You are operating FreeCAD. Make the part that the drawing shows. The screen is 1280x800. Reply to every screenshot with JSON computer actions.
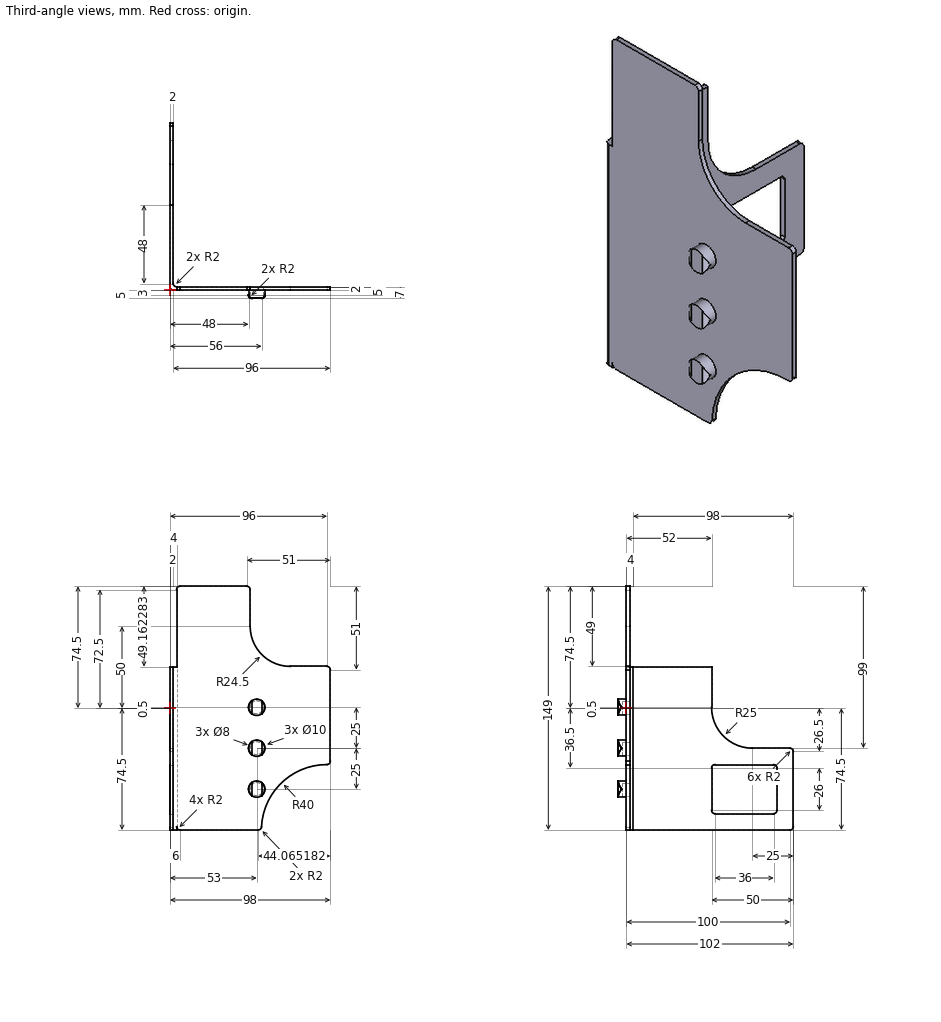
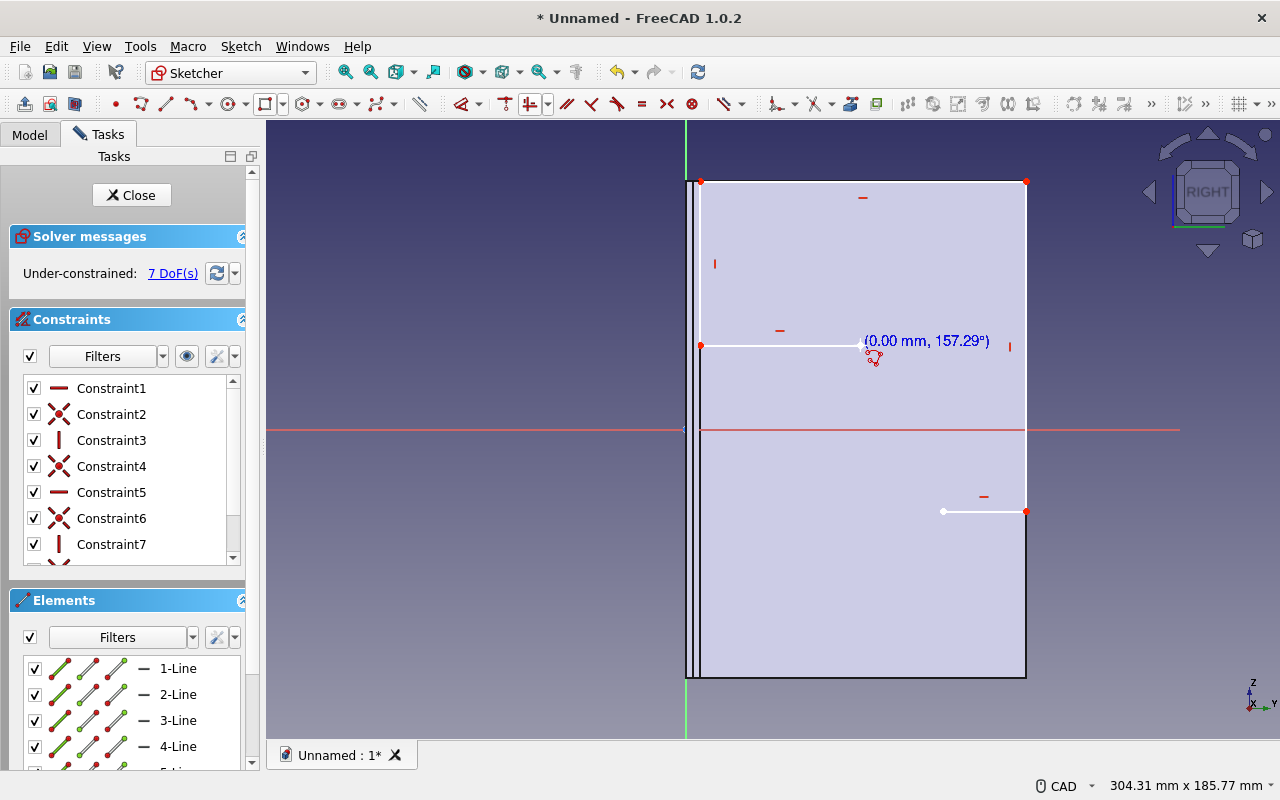
{"action": "scroll", "coordinate": [860, 428], "scroll_direction": "up", "scroll_amount": 12}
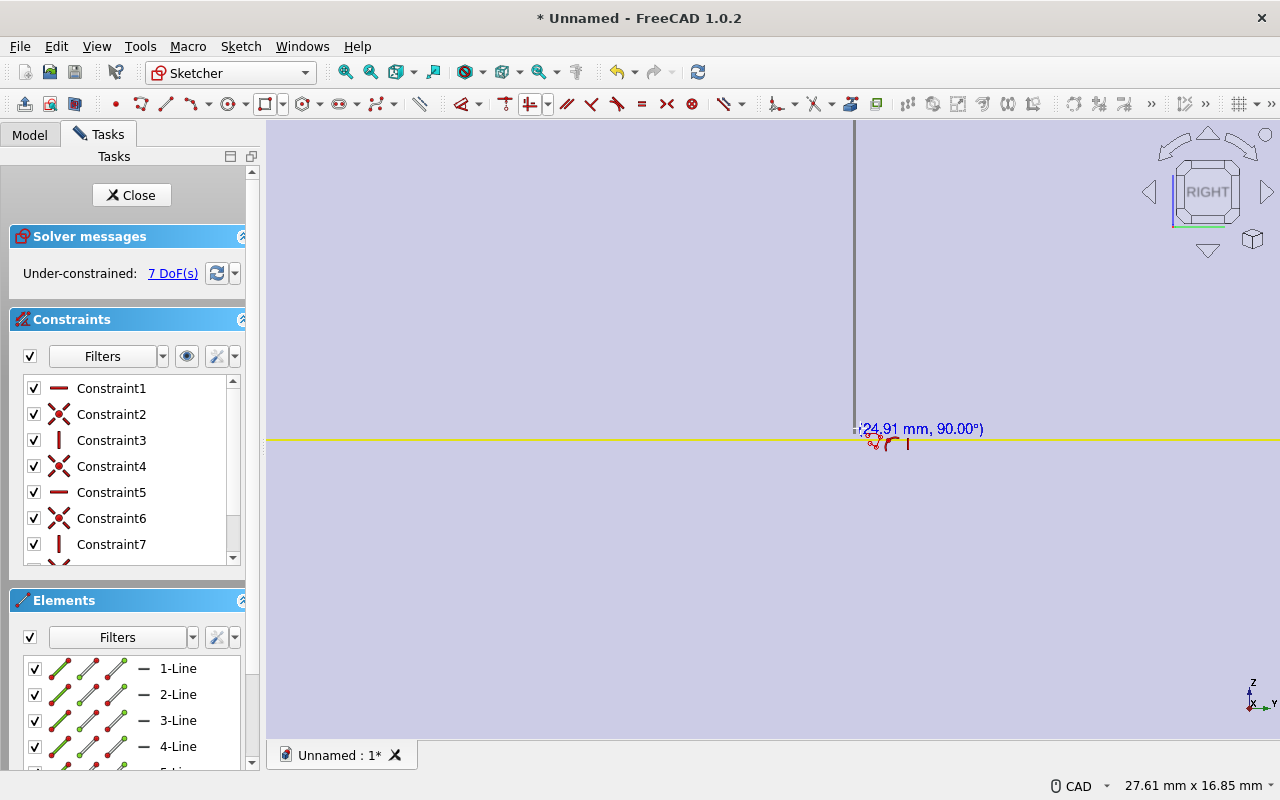
{"action": "left_click", "coordinate": [854, 421]}
{"action": "right_click", "coordinate": [854, 421]}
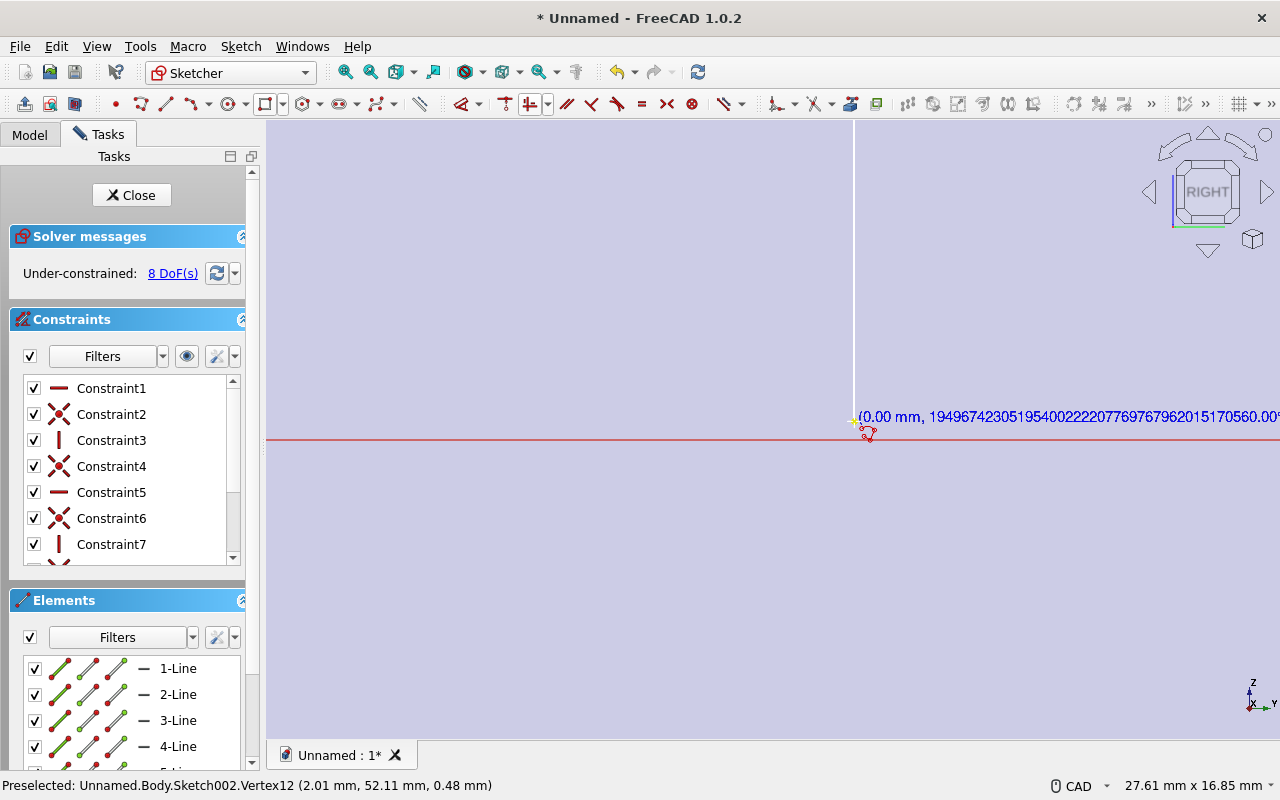
{"action": "key", "text": "g 3 a"}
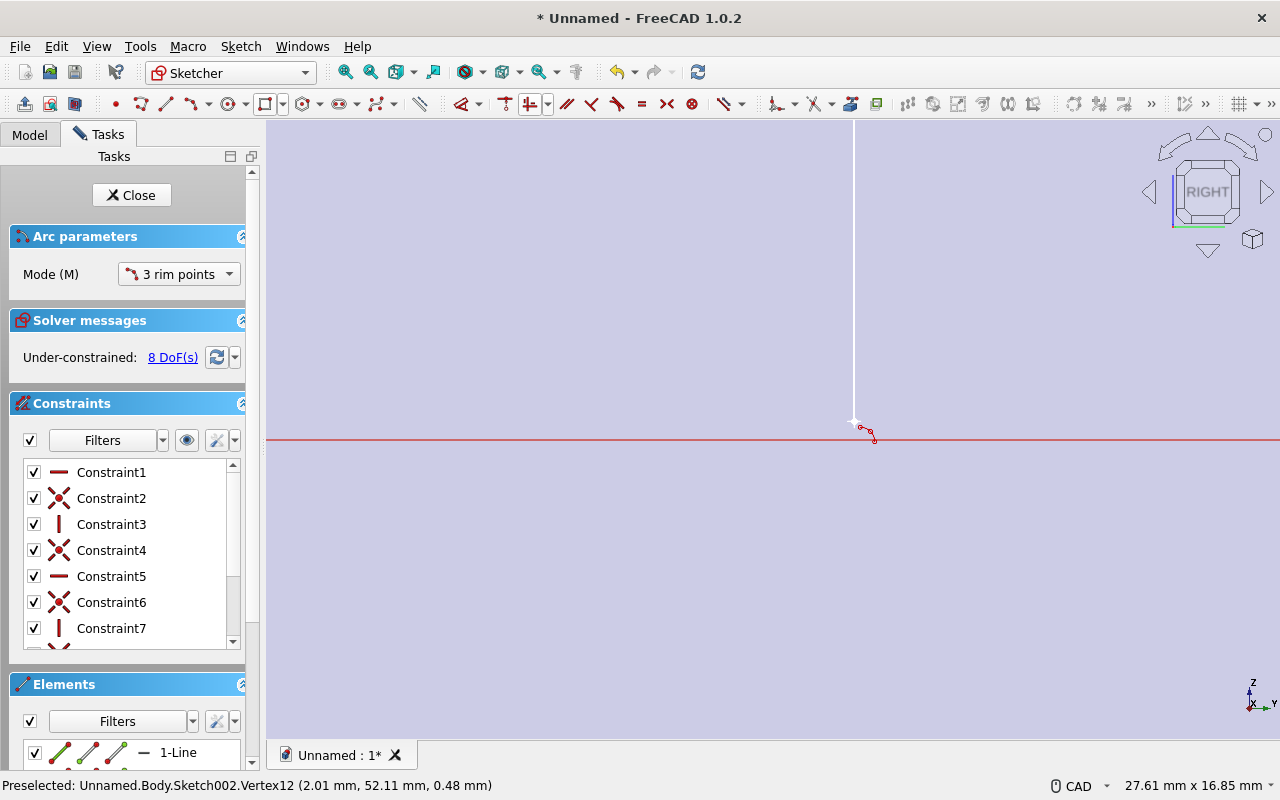
{"action": "left_click", "coordinate": [854, 422]}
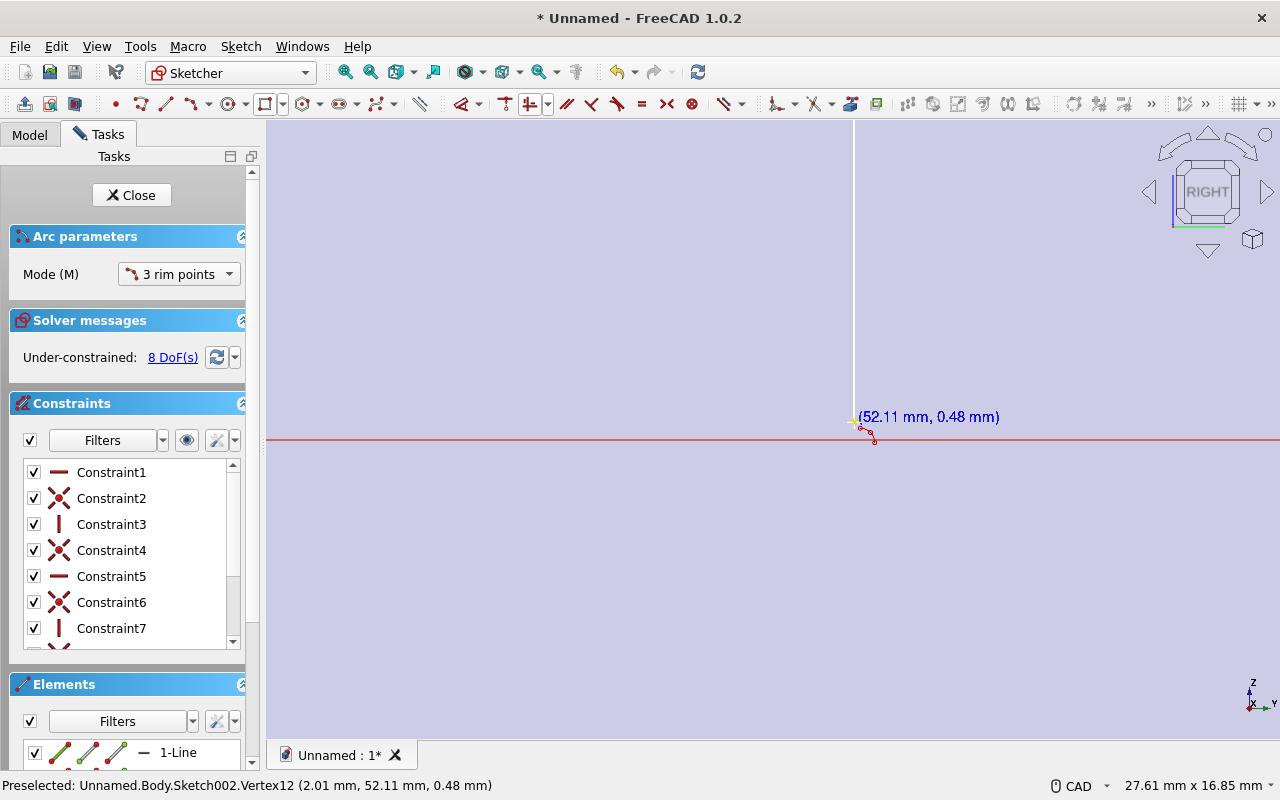
{"action": "scroll", "coordinate": [691, 543], "scroll_direction": "down", "scroll_amount": 11}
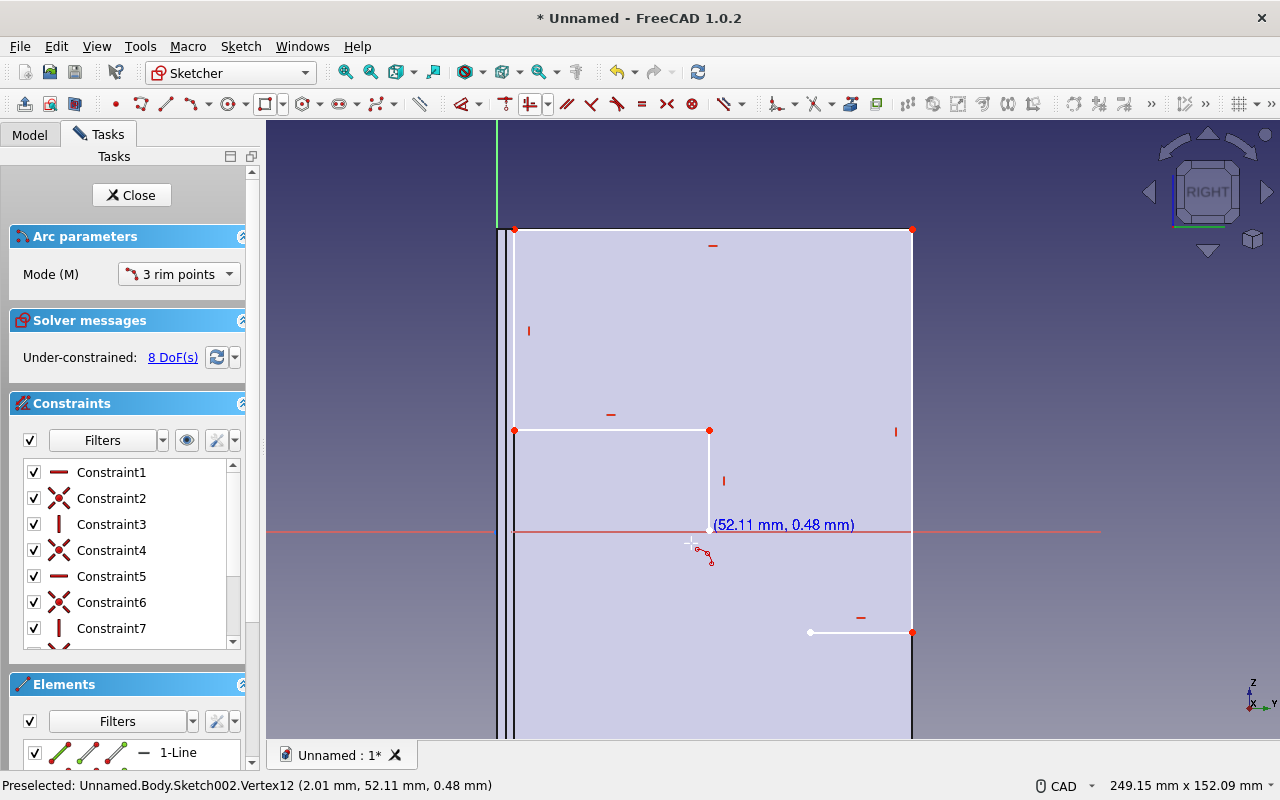
{"action": "left_click", "coordinate": [811, 633]}
{"action": "left_click", "coordinate": [739, 602]}
{"action": "key", "text": "Escape"}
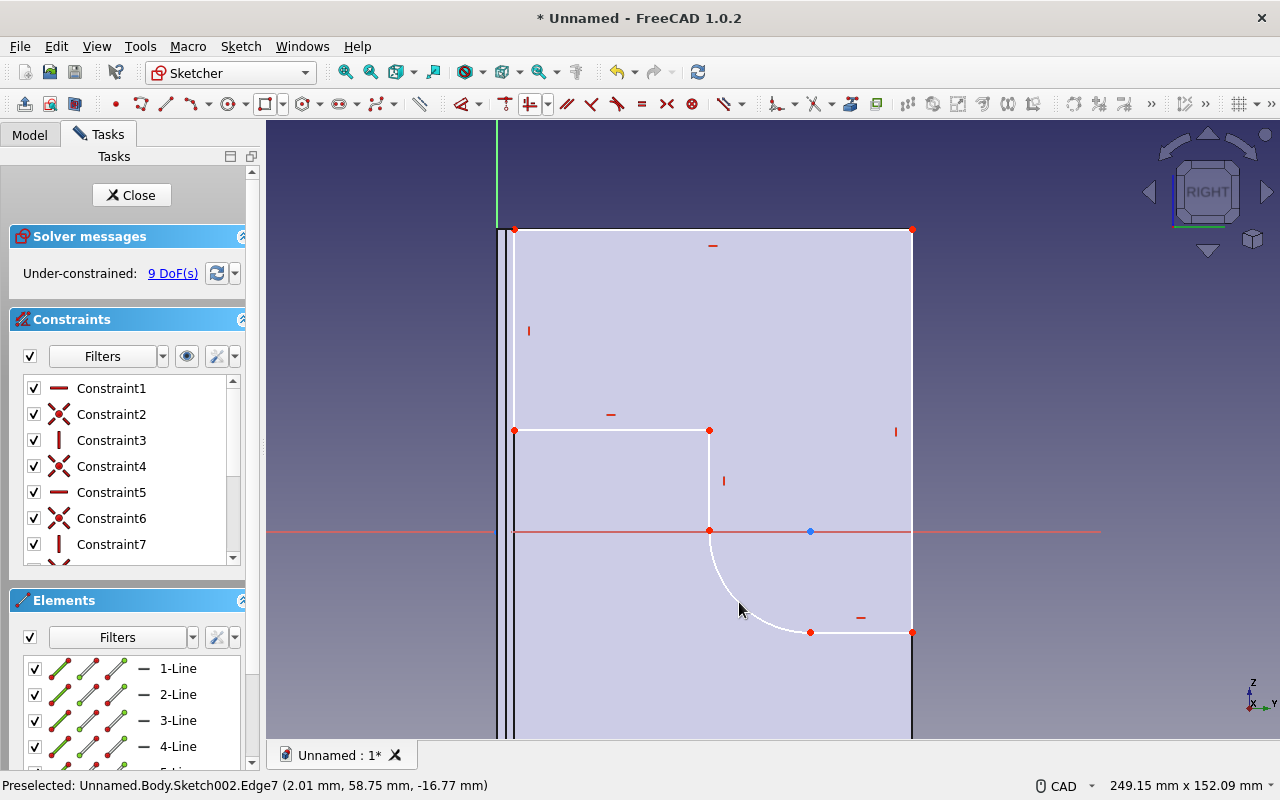
{"action": "left_click", "coordinate": [841, 633]}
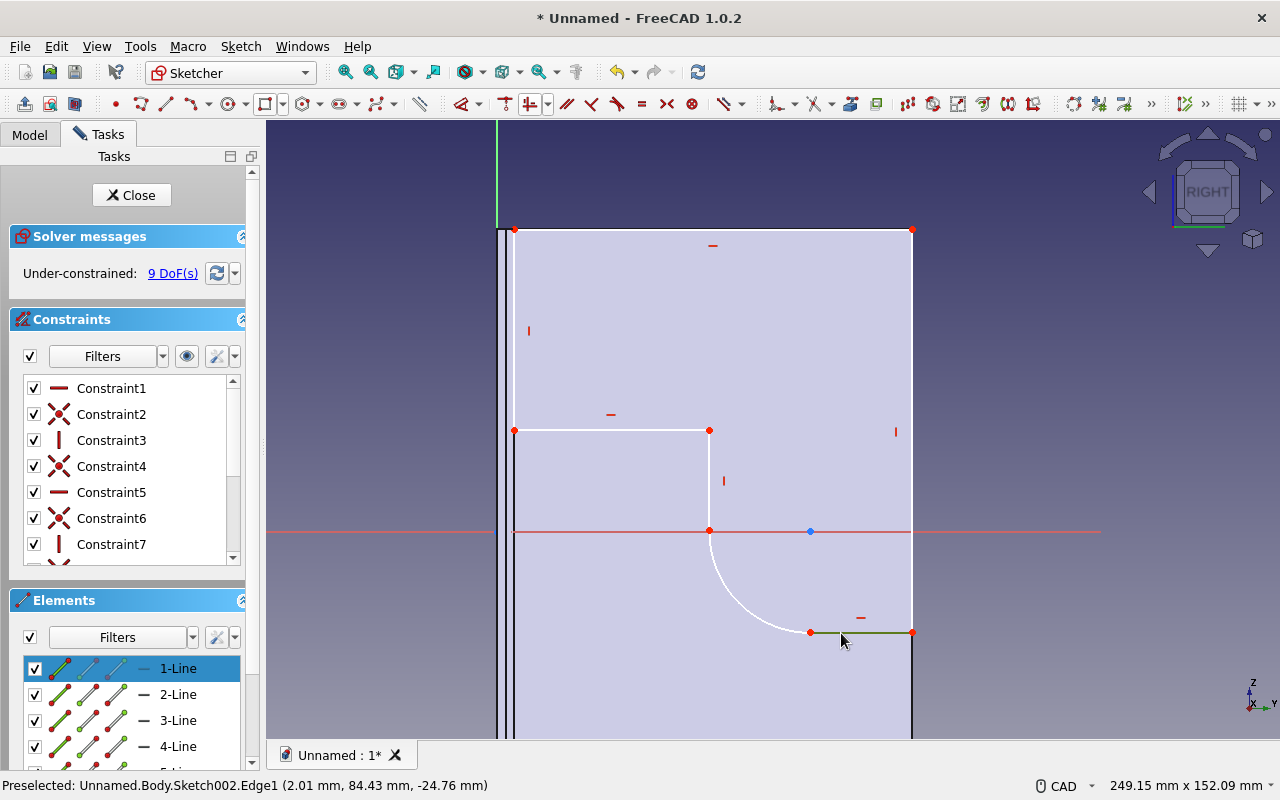
{"action": "left_click", "coordinate": [720, 577]}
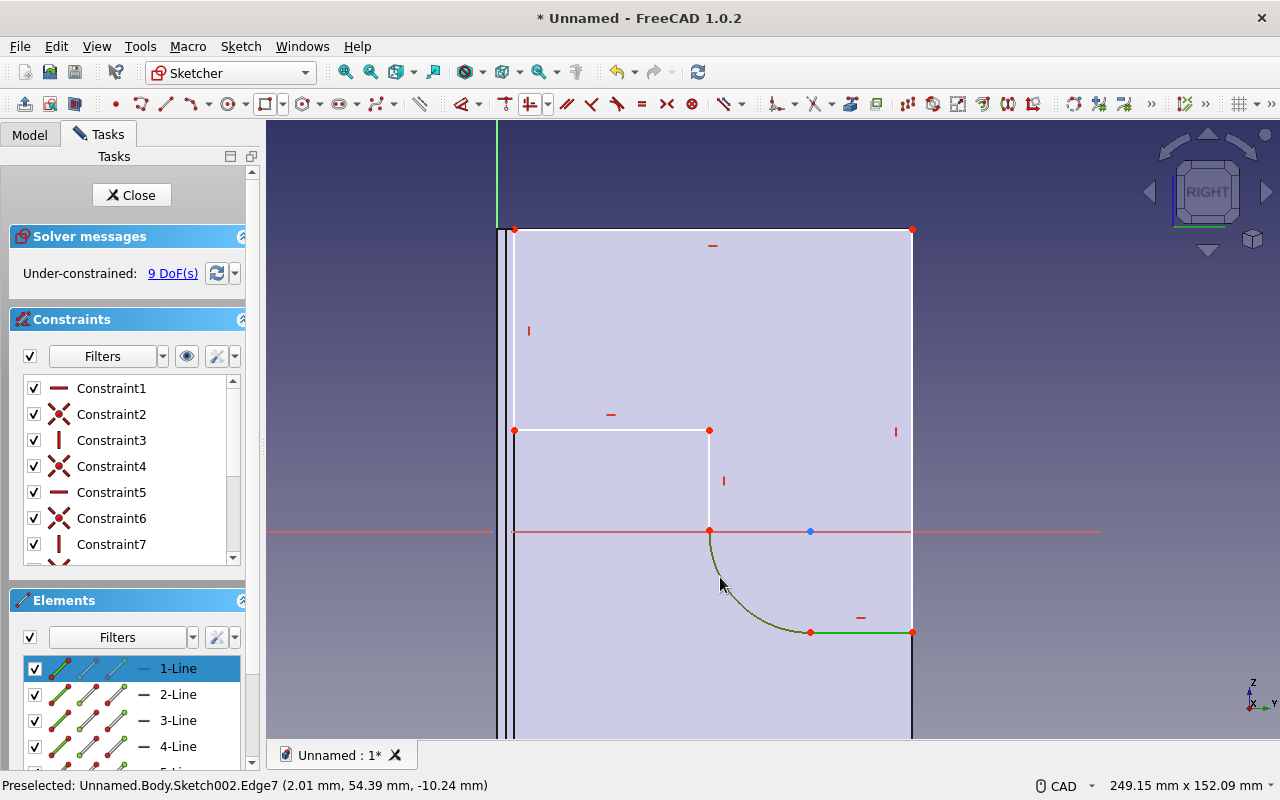
{"action": "key", "text": "t"}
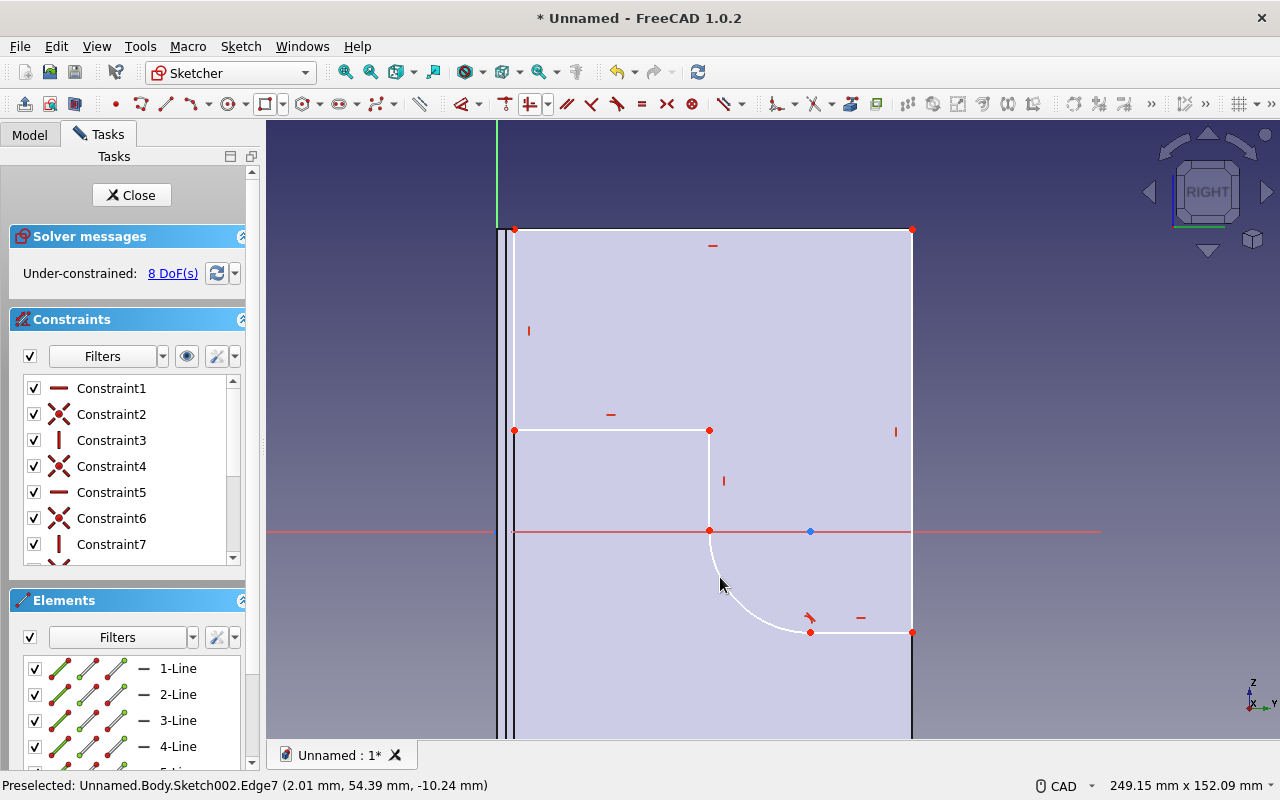
{"action": "left_click", "coordinate": [709, 460]}